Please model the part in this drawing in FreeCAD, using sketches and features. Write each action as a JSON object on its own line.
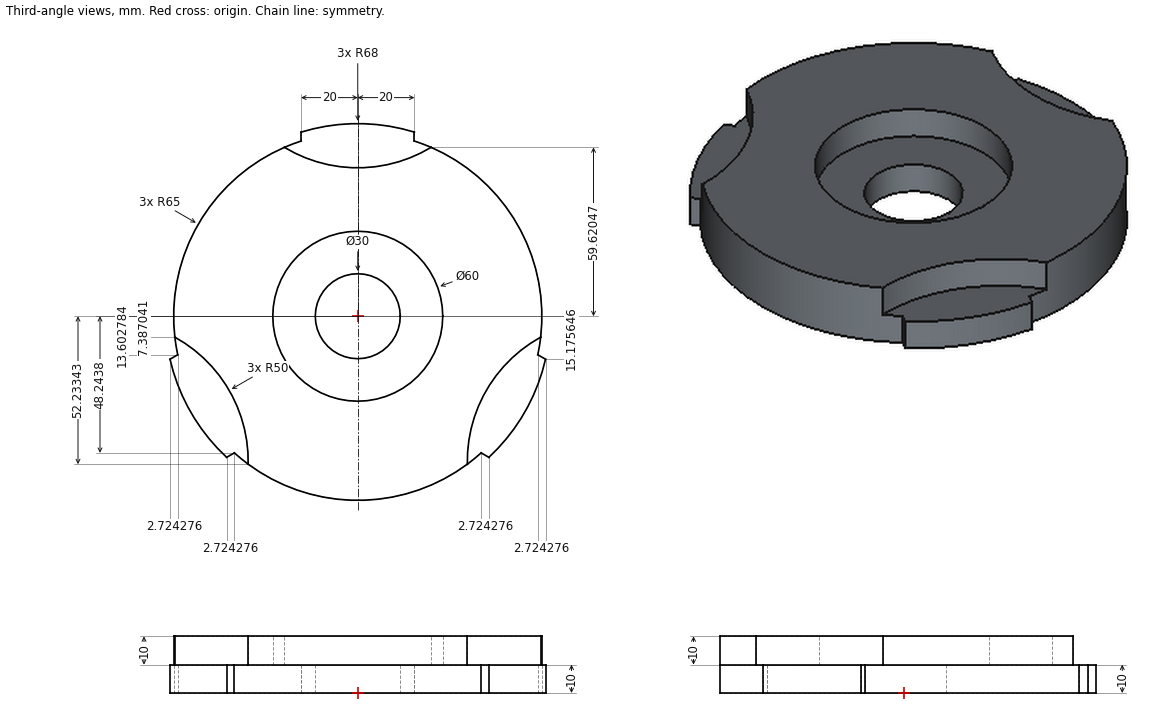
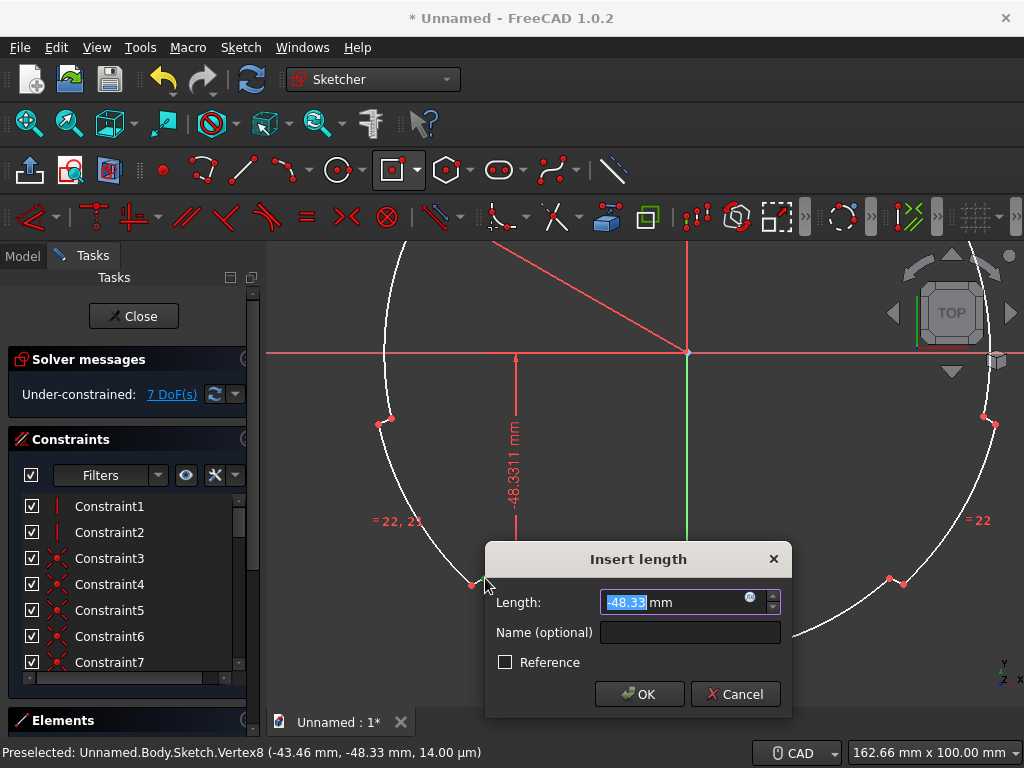
{"action": "type", "text": "-48.2438"}
{"action": "key", "text": "Return"}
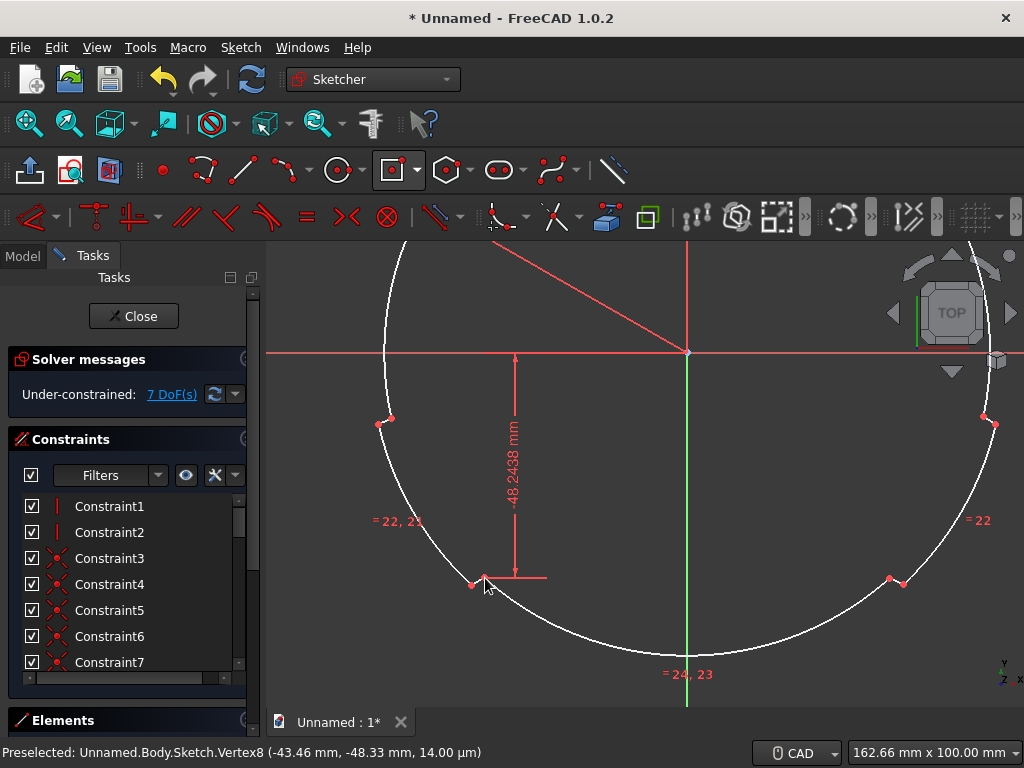
{"action": "scroll", "coordinate": [486, 579], "scroll_direction": "down", "scroll_amount": 4}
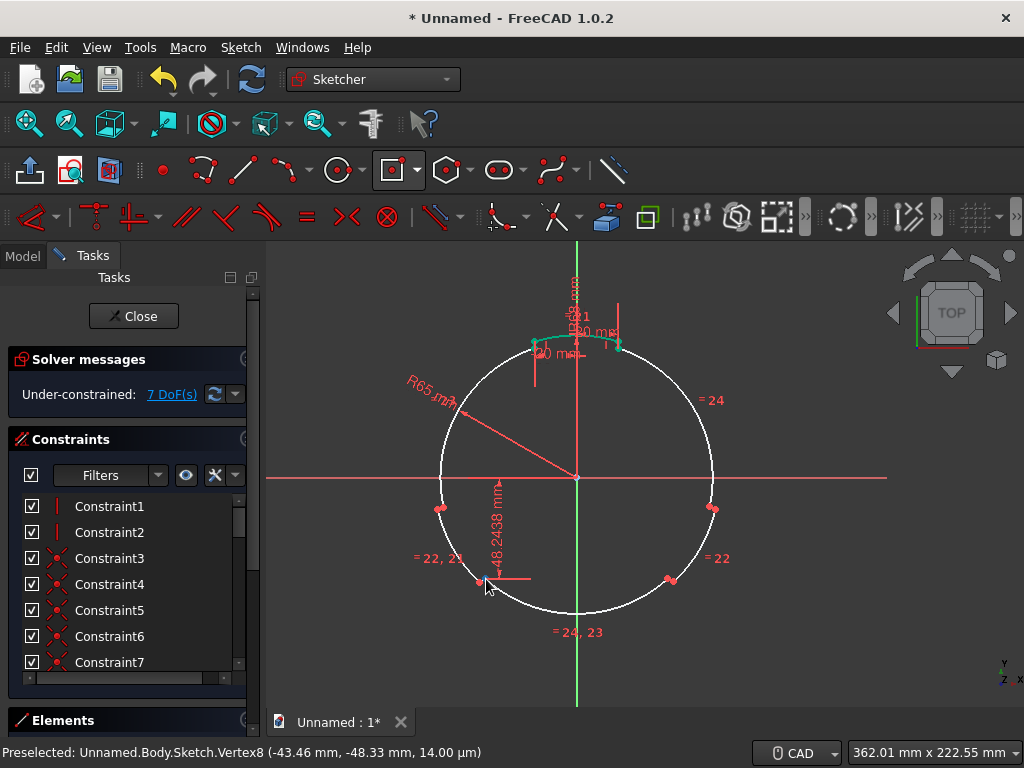
{"action": "scroll", "coordinate": [668, 579], "scroll_direction": "up", "scroll_amount": 3}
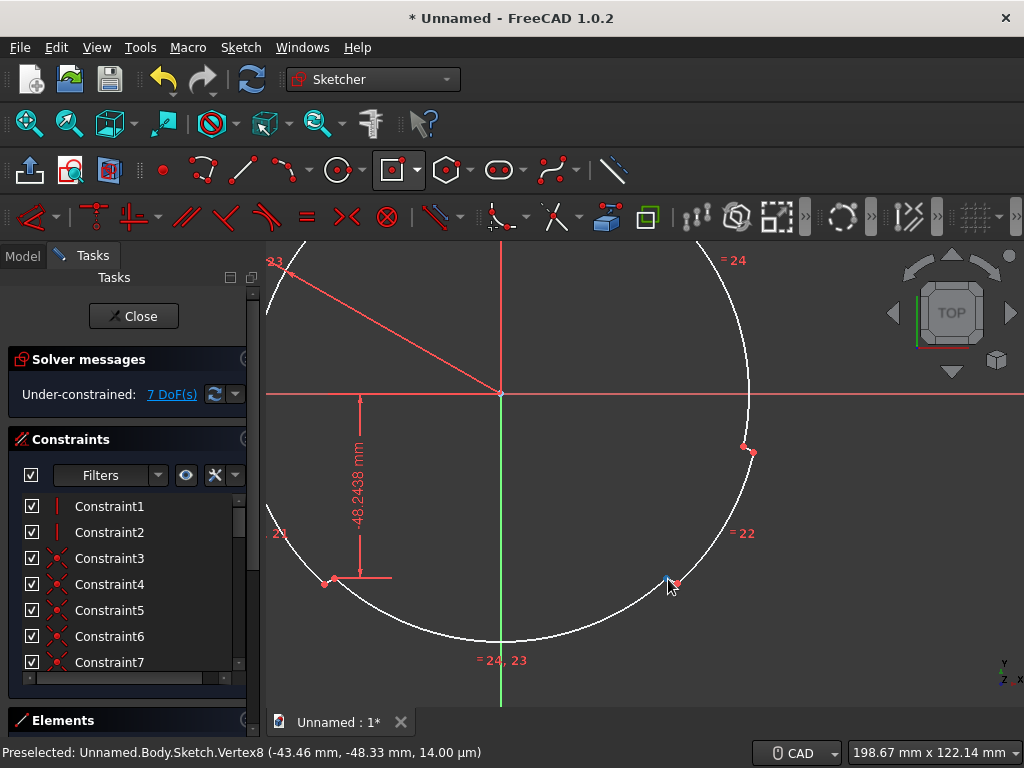
{"action": "left_click", "coordinate": [667, 578]}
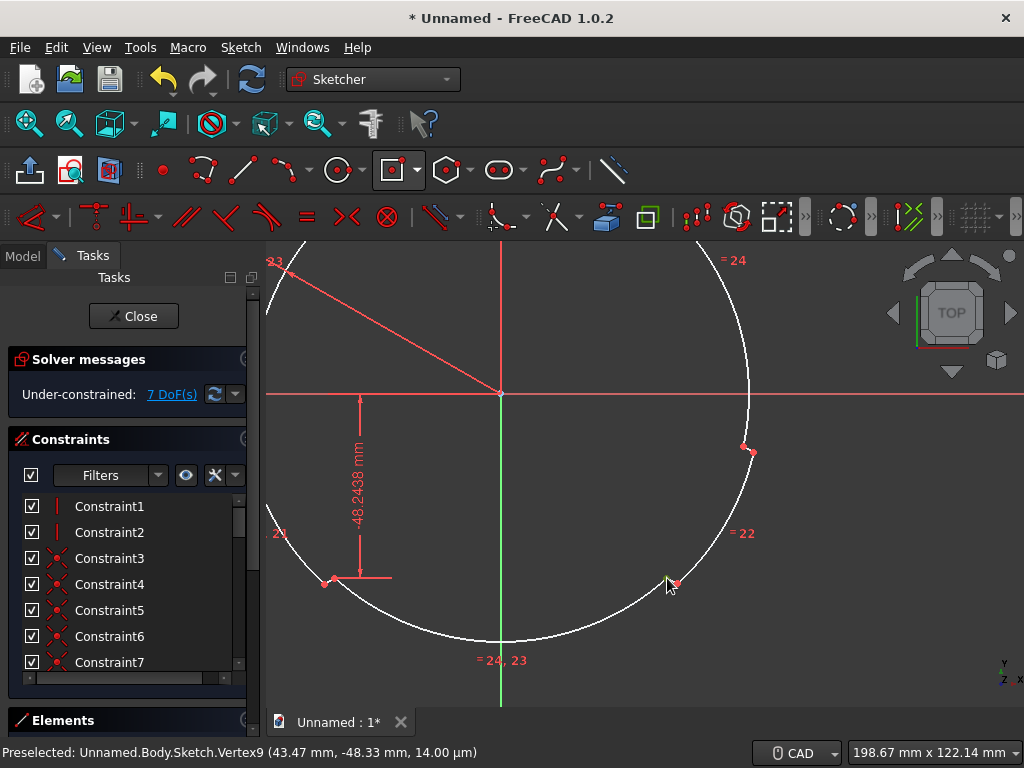
{"action": "left_click", "coordinate": [58, 218]}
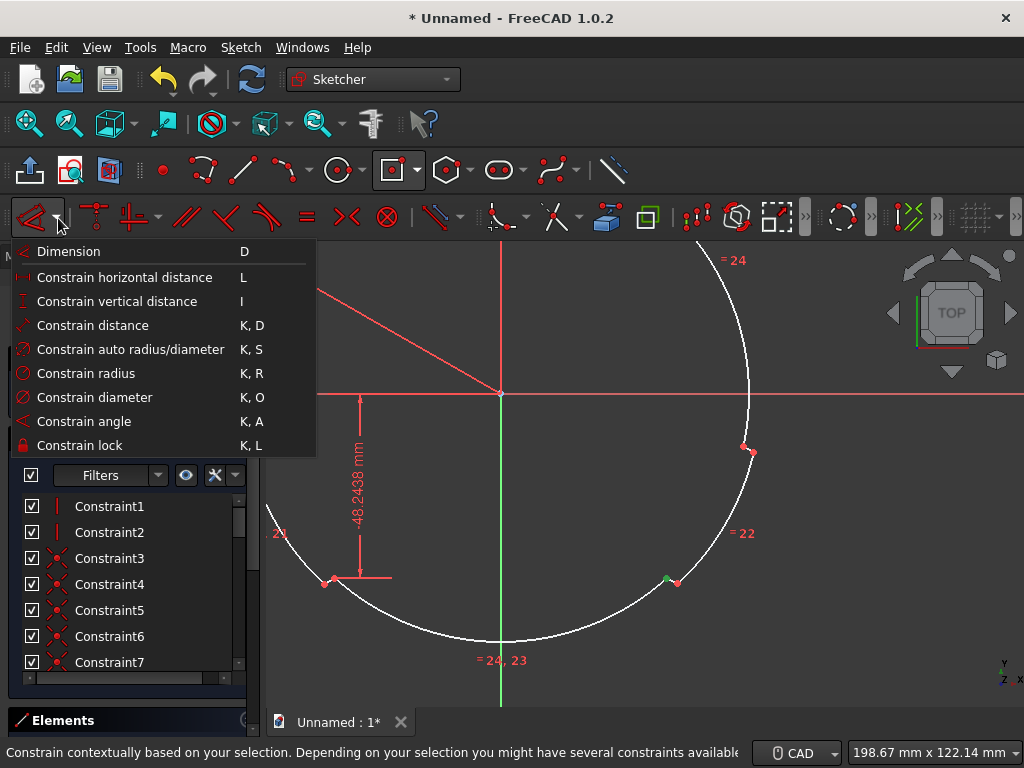
{"action": "left_click", "coordinate": [164, 301]}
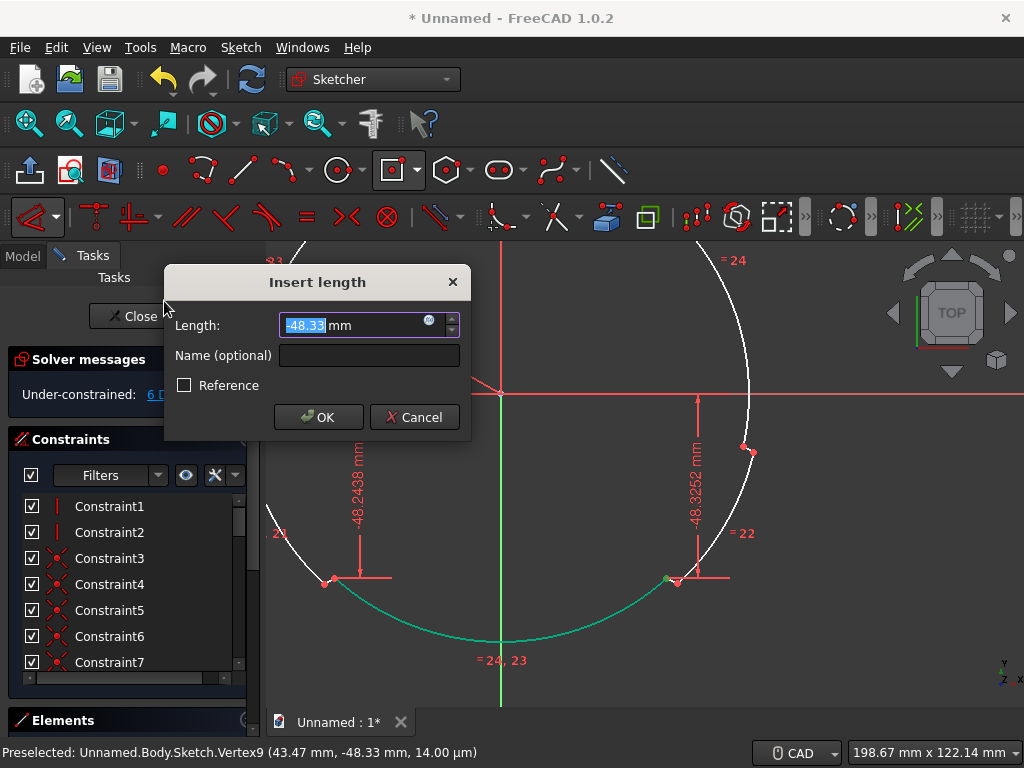
{"action": "type", "text": "-48.2438"}
{"action": "key", "text": "Return"}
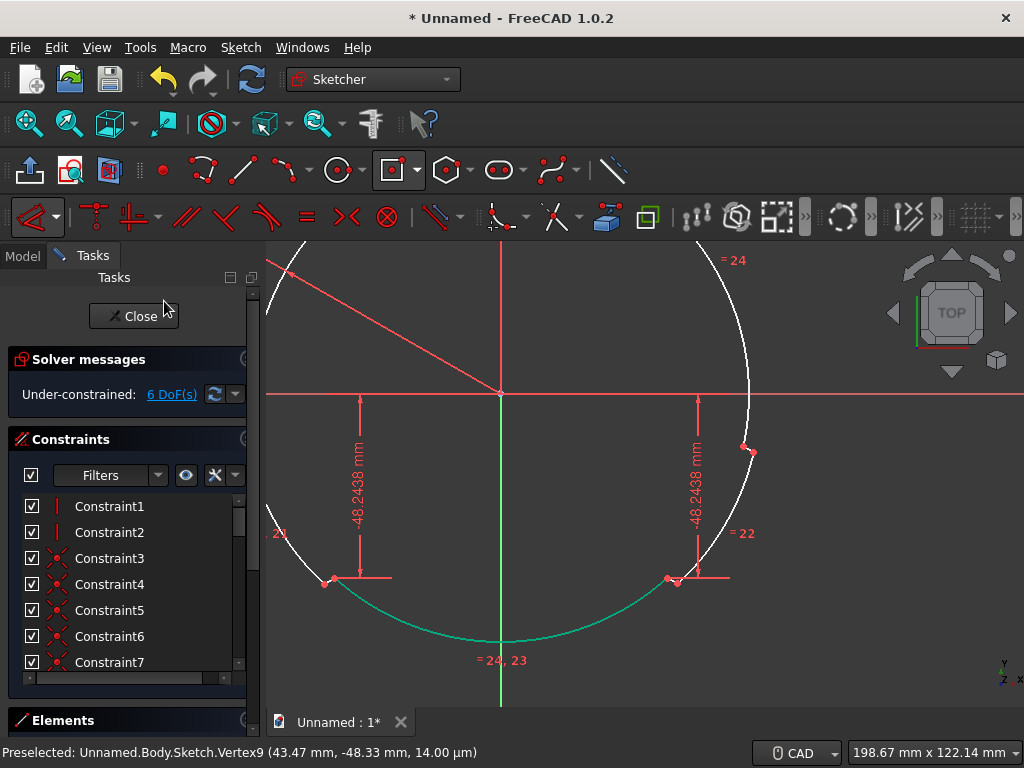
{"action": "scroll", "coordinate": [668, 578], "scroll_direction": "down", "scroll_amount": 3}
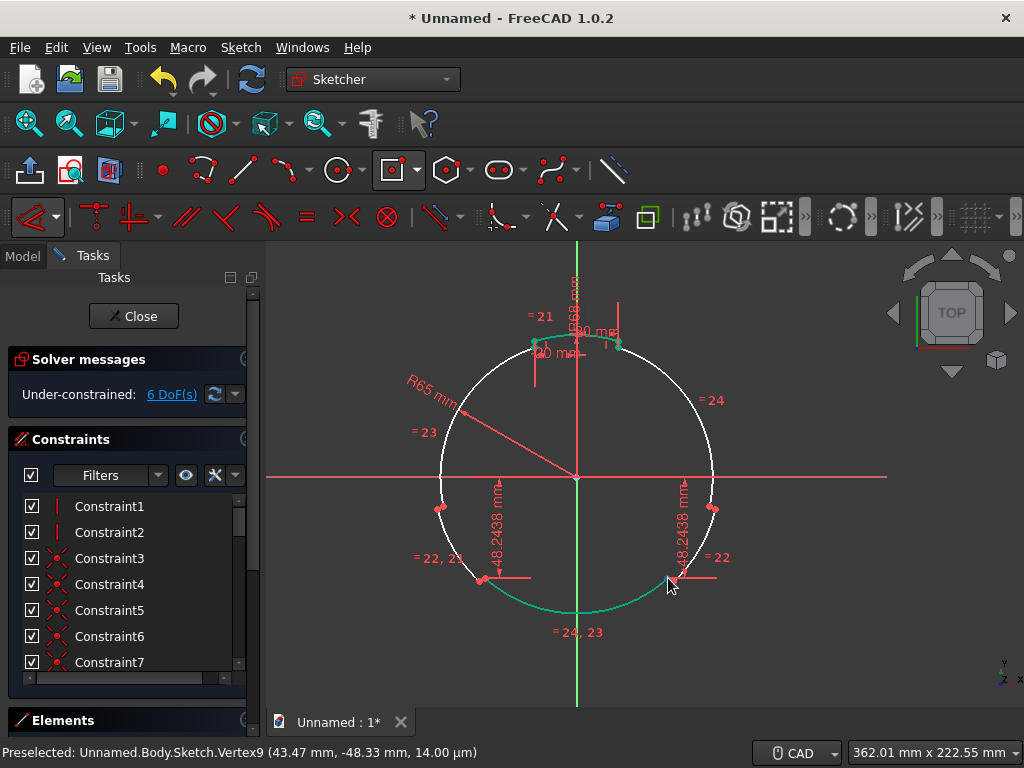
{"action": "scroll", "coordinate": [441, 508], "scroll_direction": "up", "scroll_amount": 10}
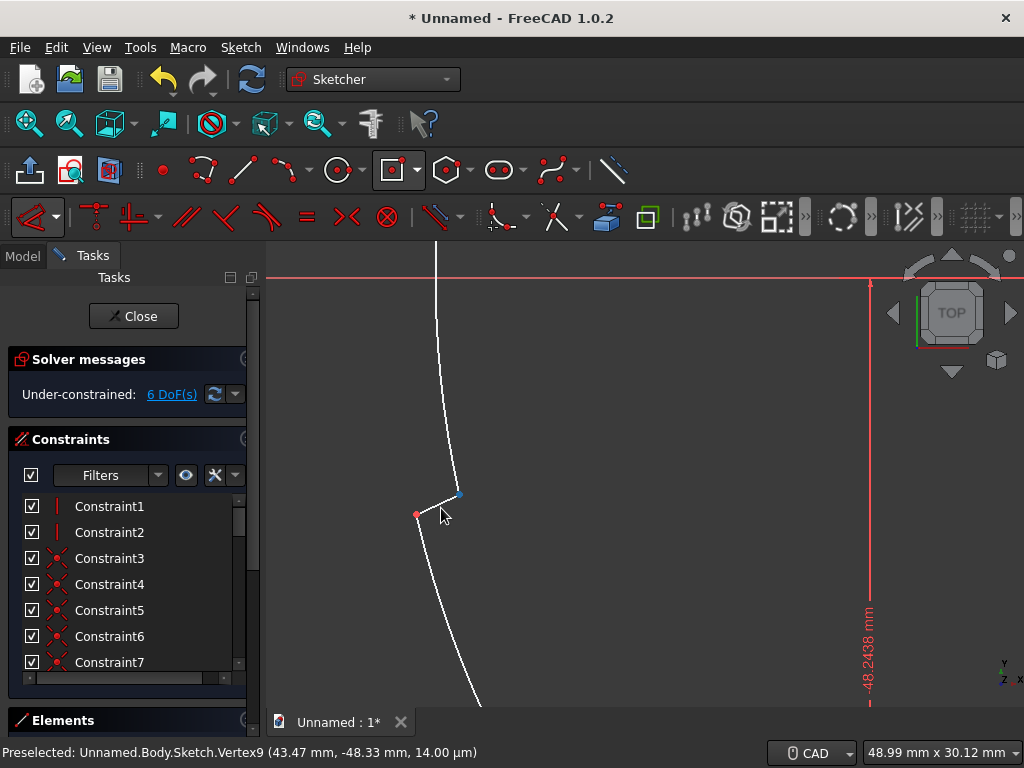
{"action": "left_click", "coordinate": [438, 505]}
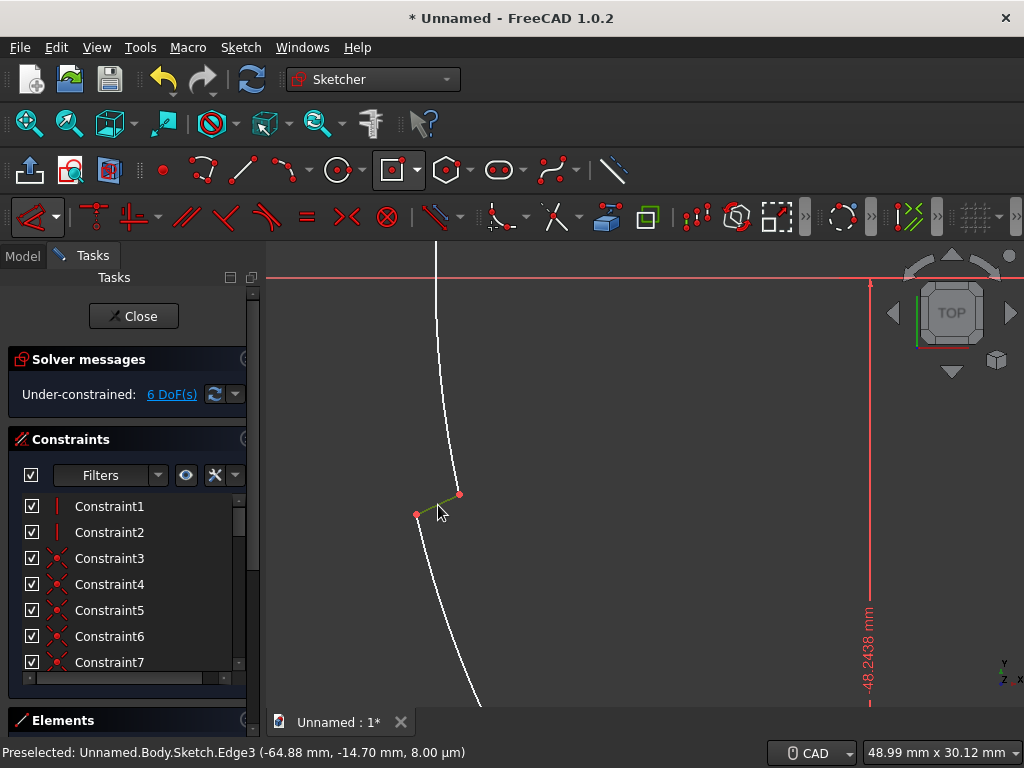
{"action": "left_click", "coordinate": [58, 218]}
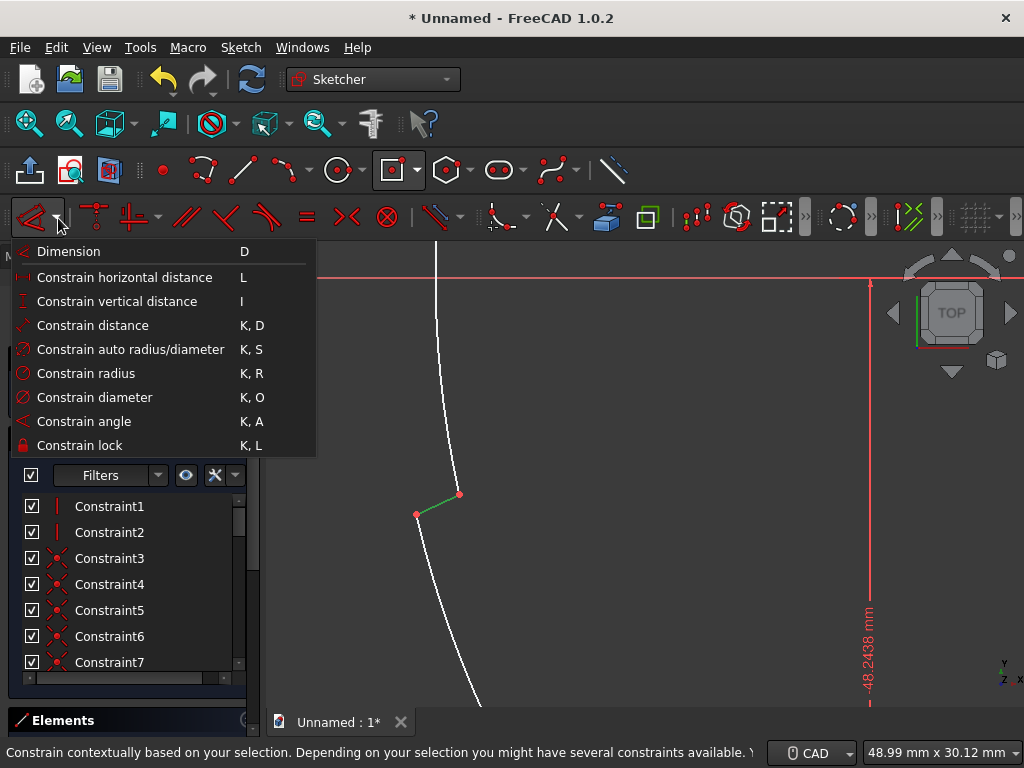
{"action": "left_click", "coordinate": [164, 277]}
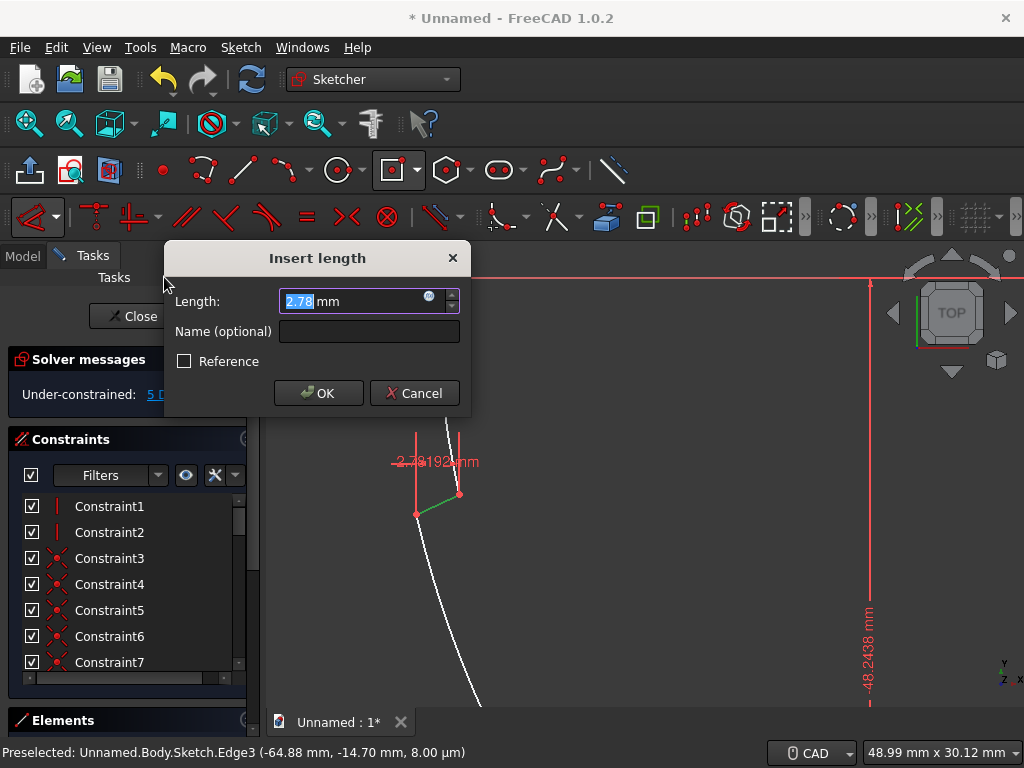
{"action": "type", "text": "2.724276"}
{"action": "key", "text": "Return"}